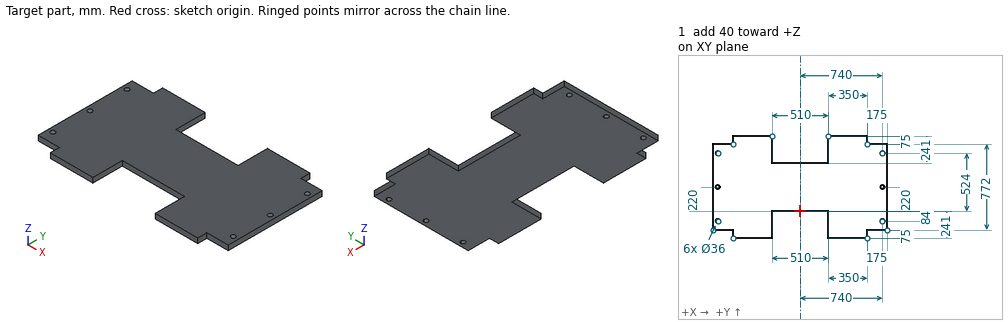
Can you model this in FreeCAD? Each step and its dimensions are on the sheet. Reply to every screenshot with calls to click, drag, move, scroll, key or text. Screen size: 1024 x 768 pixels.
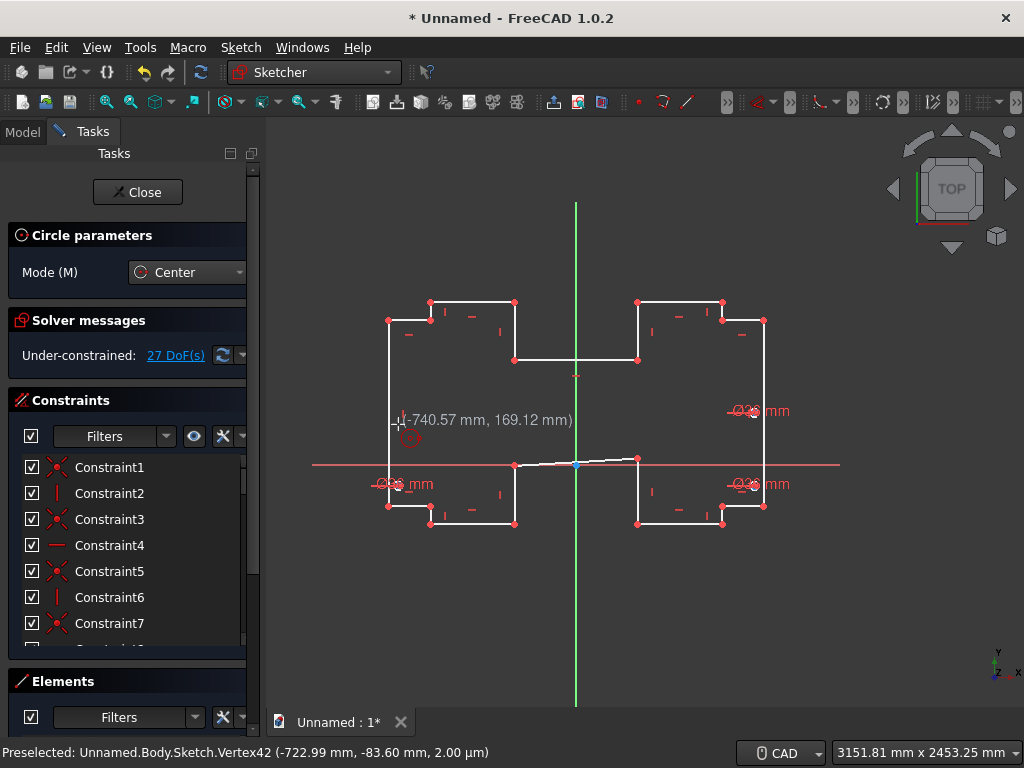
scroll(398, 412, up, 3)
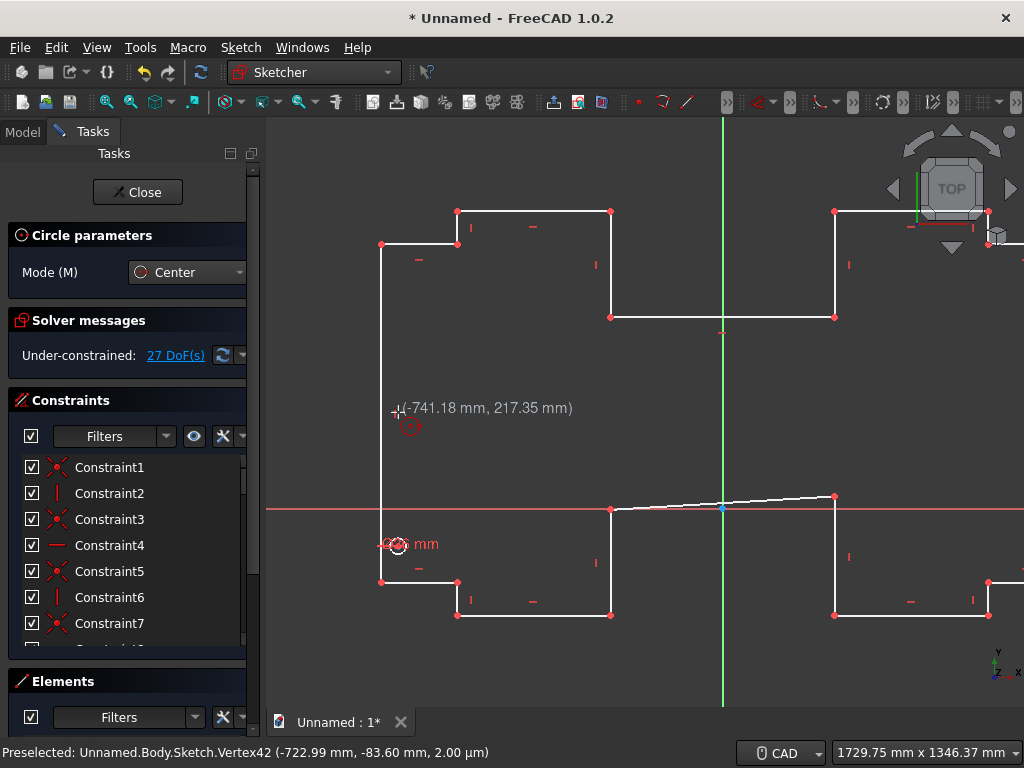
click(398, 412)
move(404, 407)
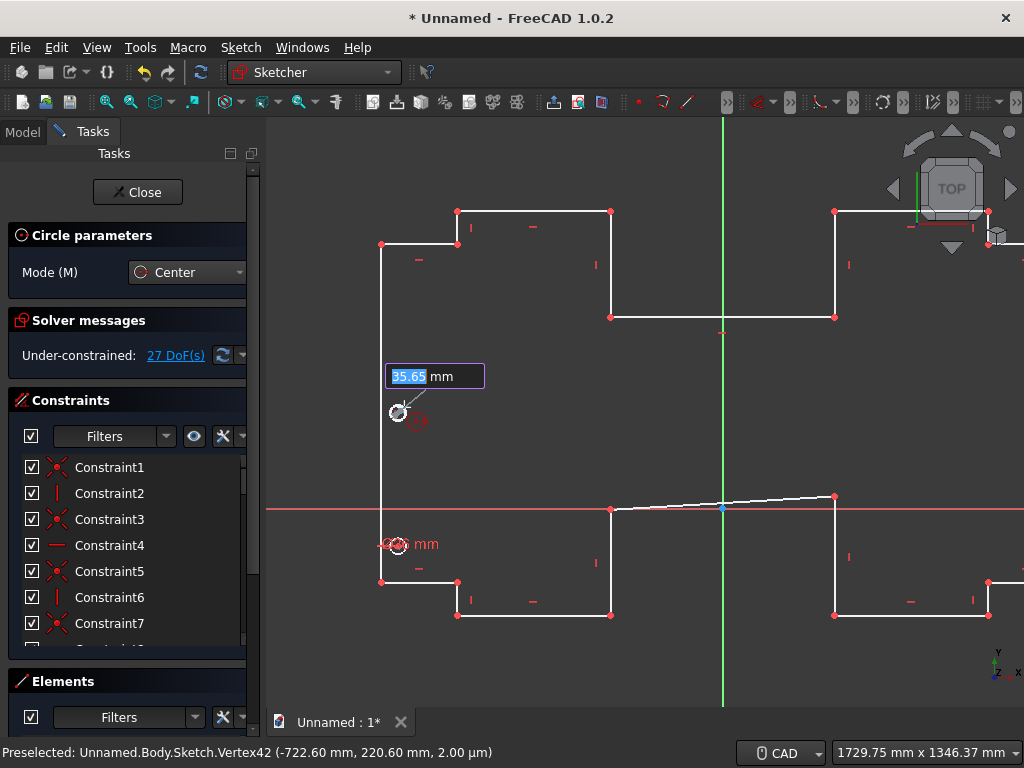
text(36)
key(Return)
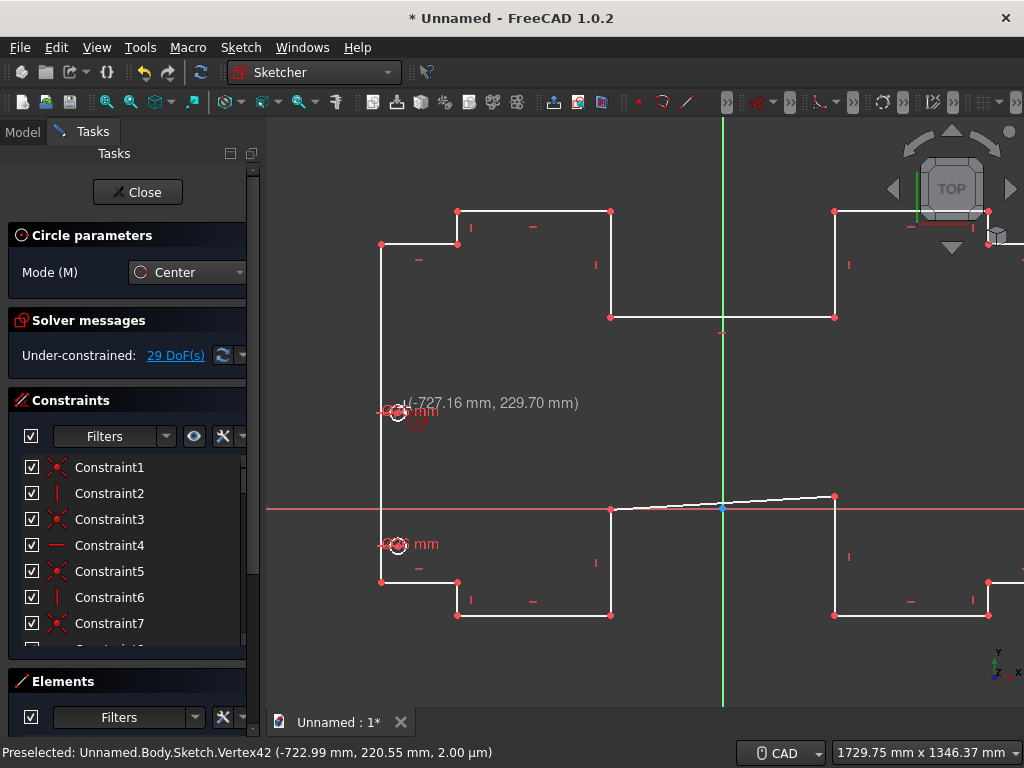
scroll(399, 412, down, 3)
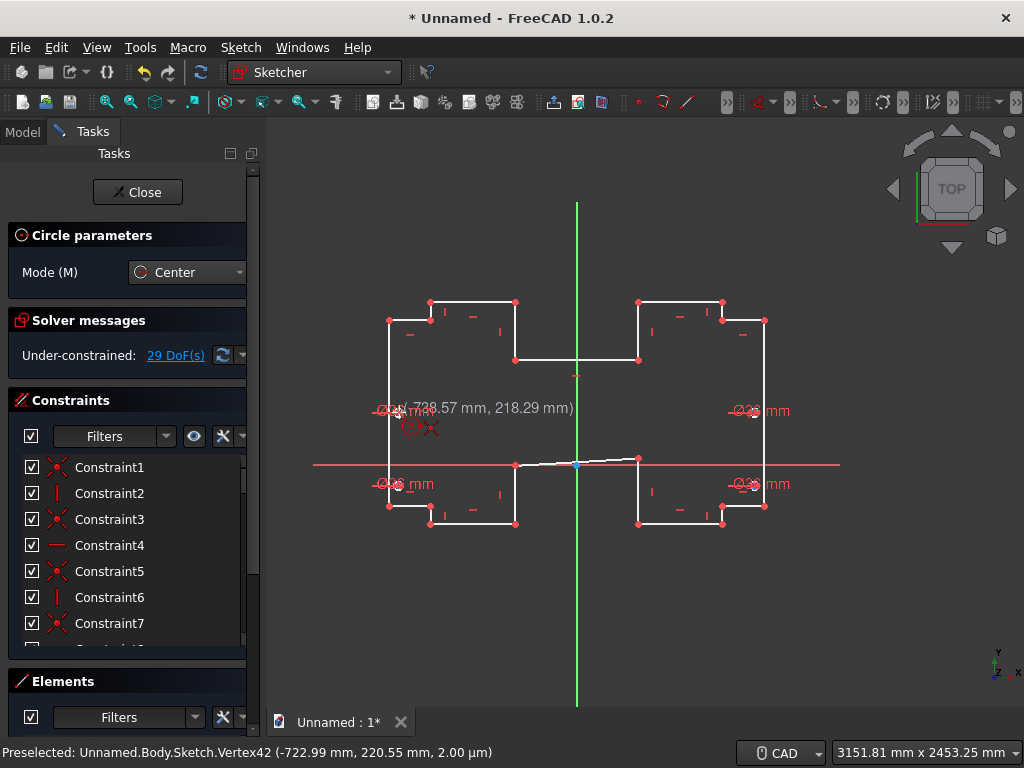
scroll(755, 339, up, 9)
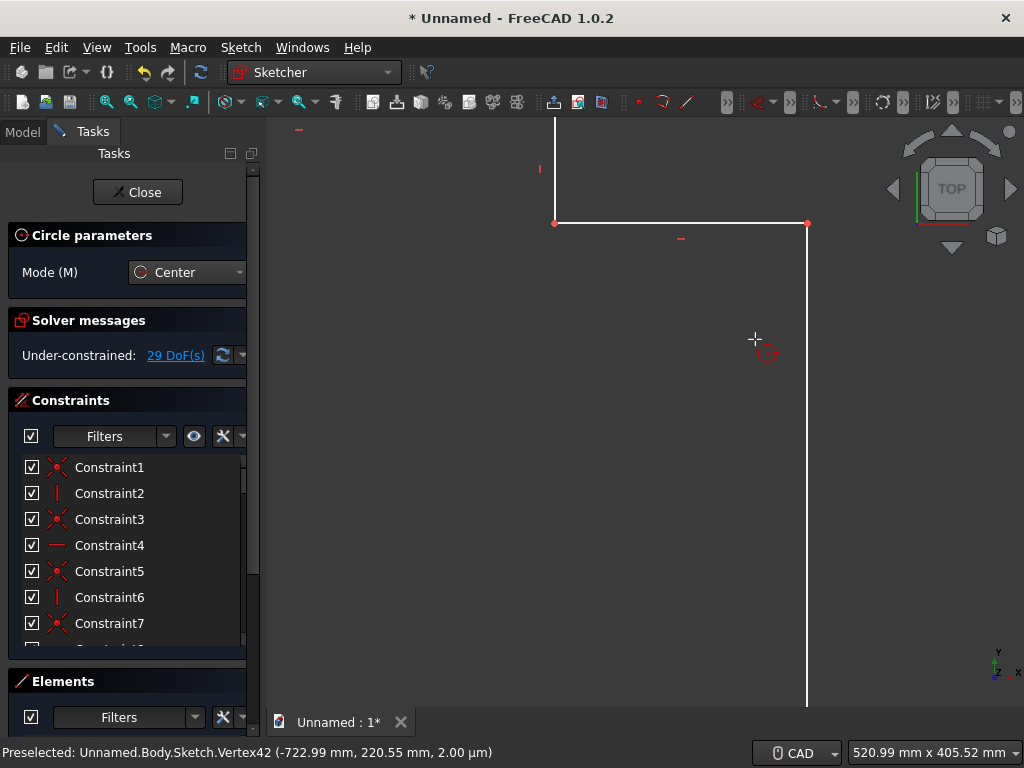
scroll(755, 339, down, 9)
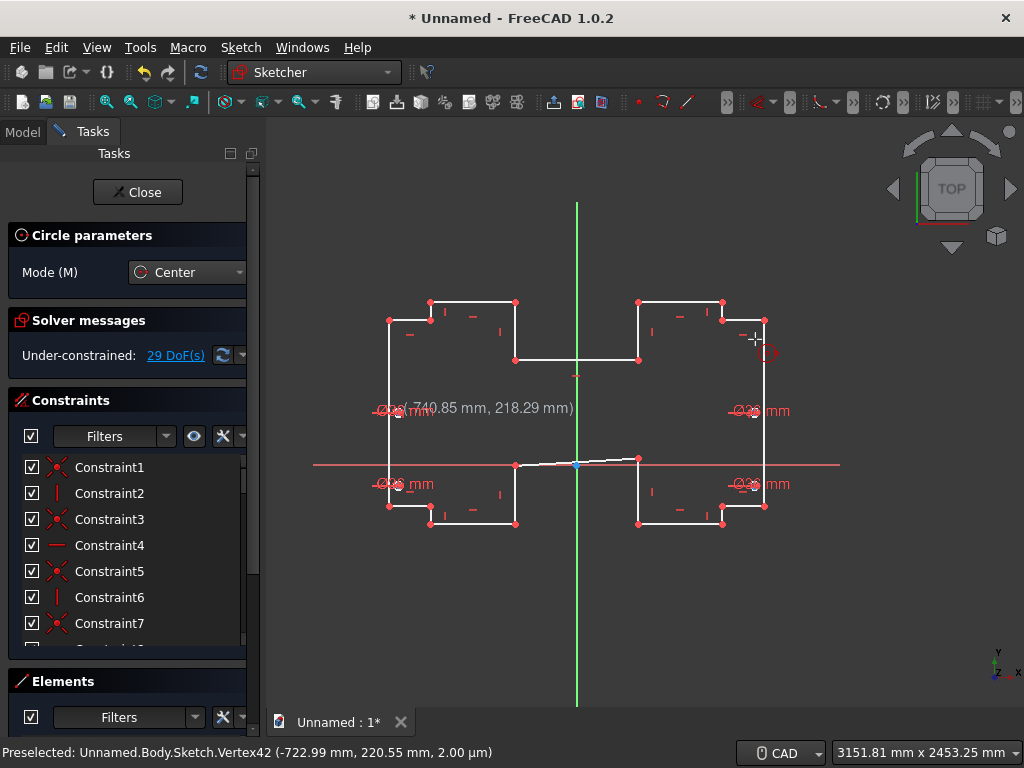
scroll(755, 339, up, 3)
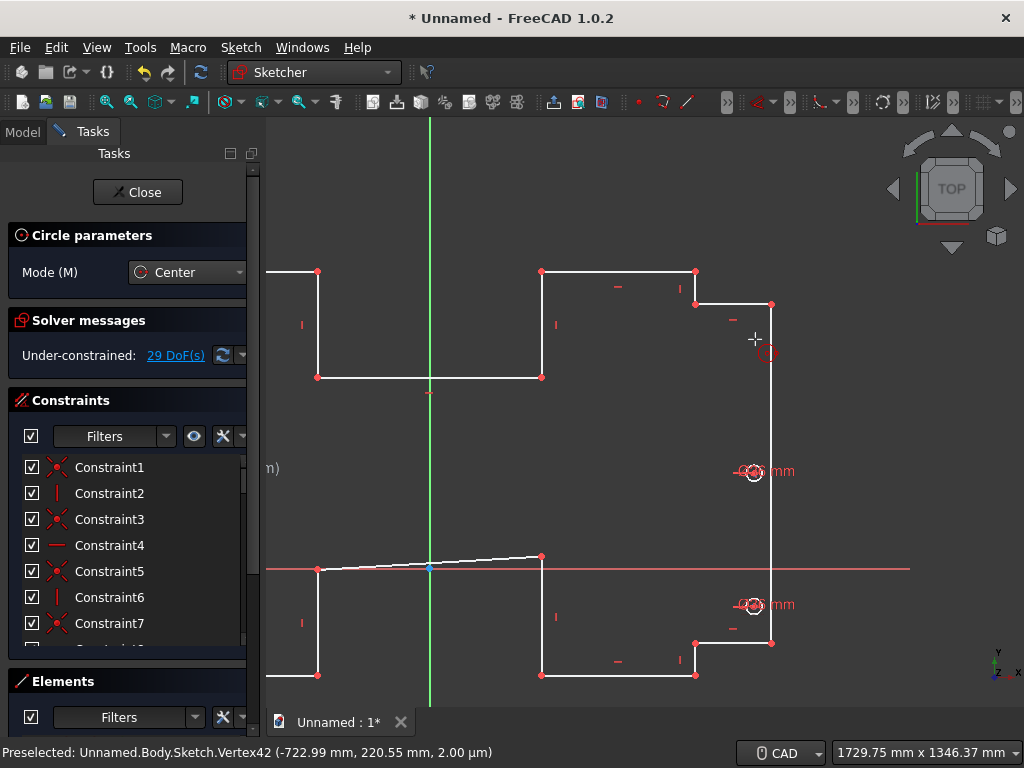
click(754, 339)
move(748, 334)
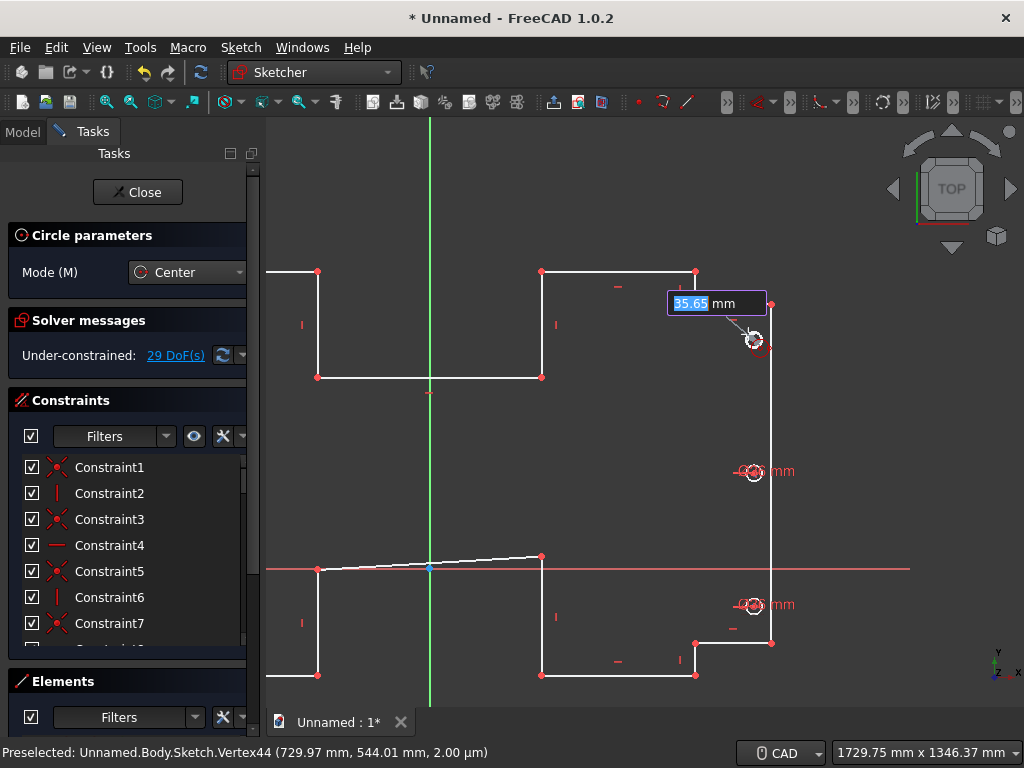
text(36)
key(Return)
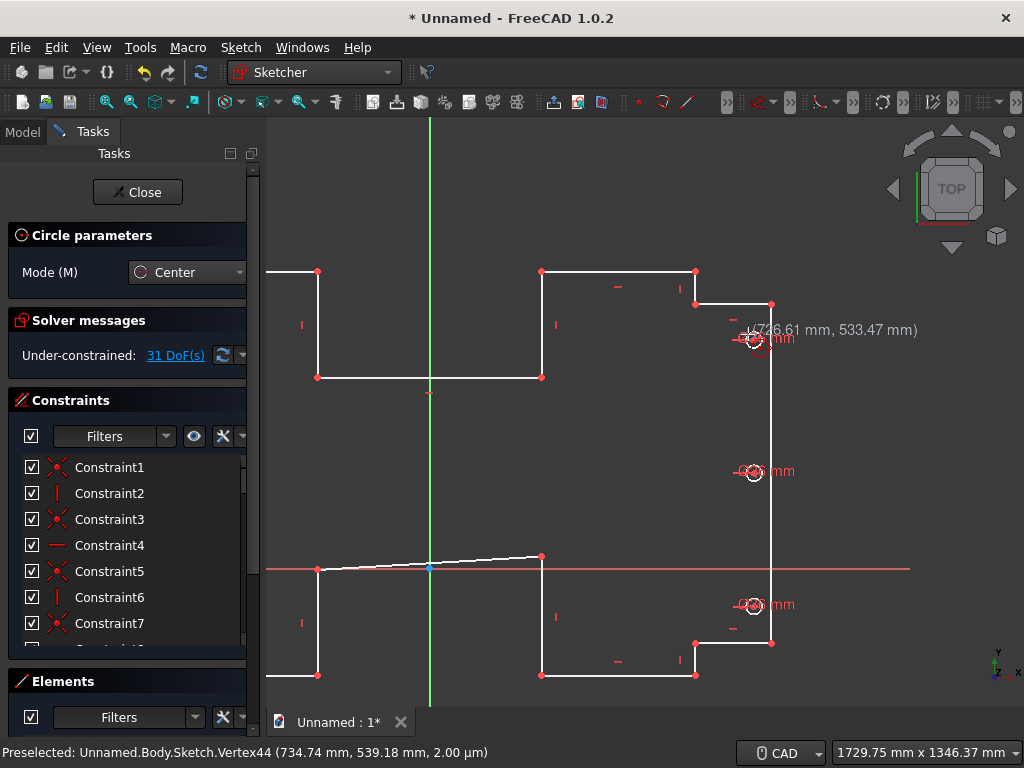
scroll(755, 339, down, 3)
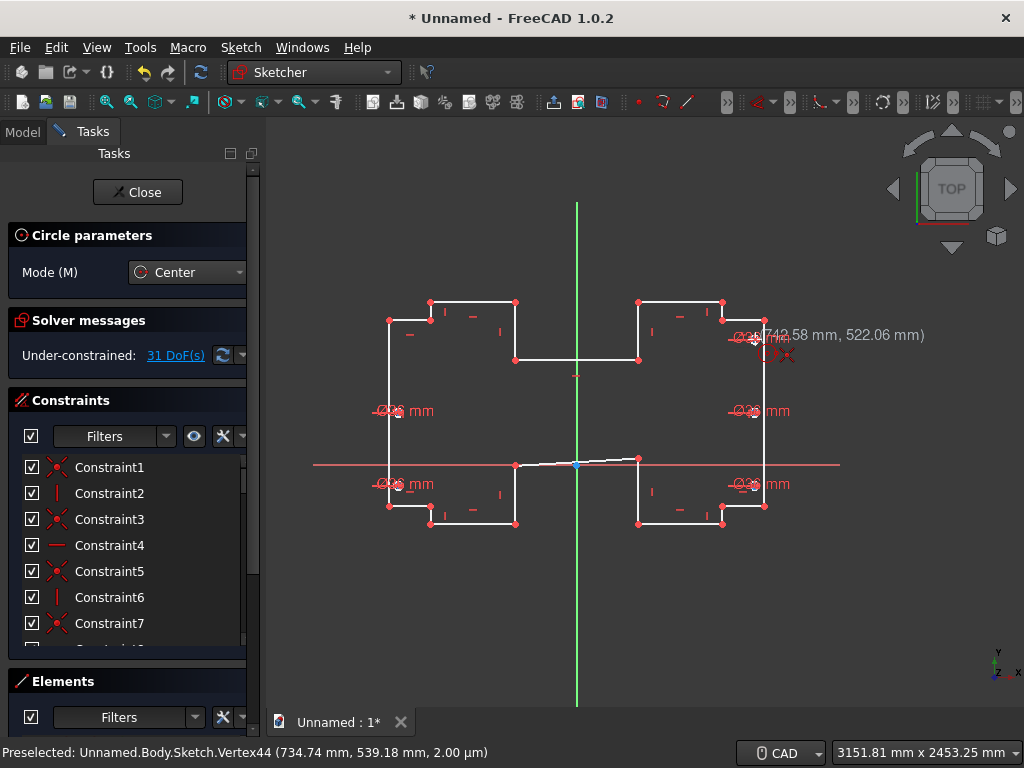
scroll(399, 339, up, 9)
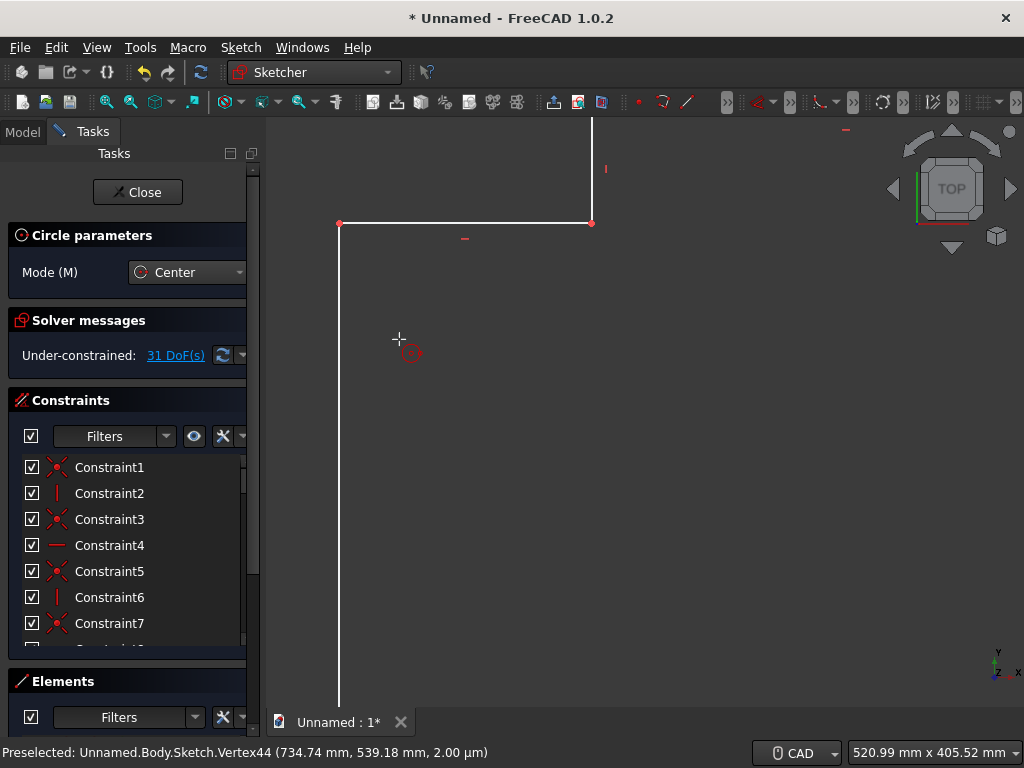
scroll(399, 339, down, 9)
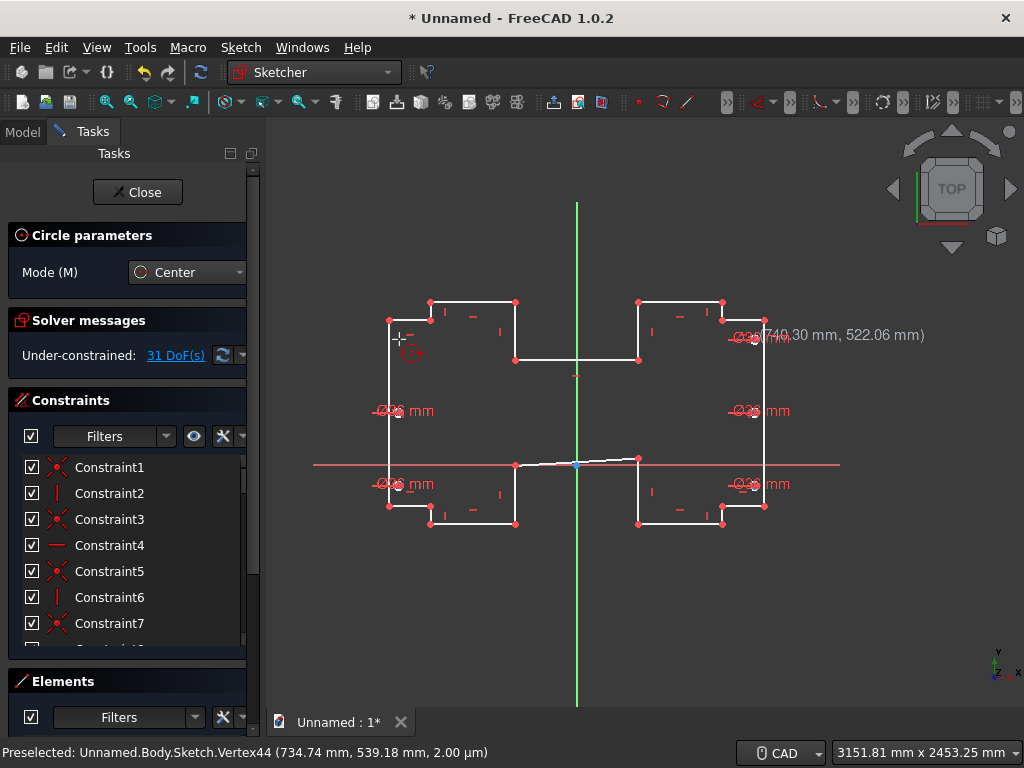
scroll(399, 339, up, 3)